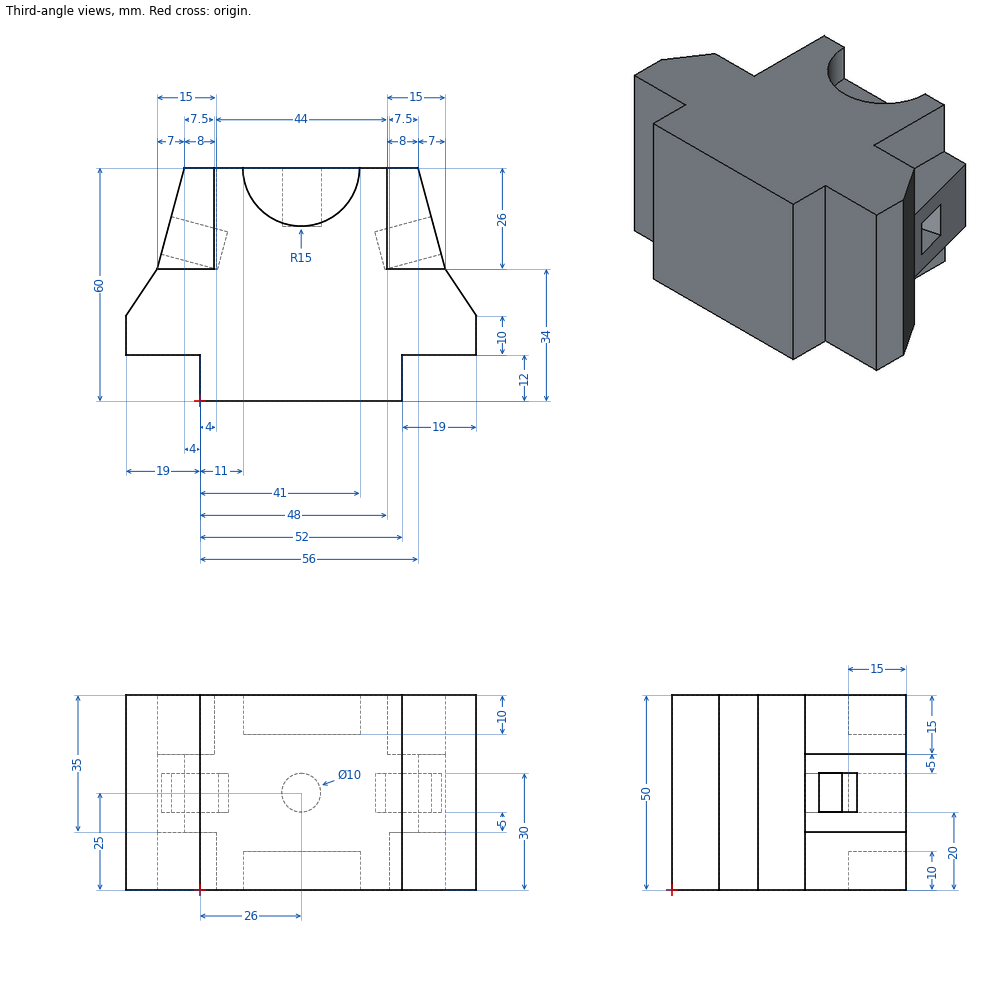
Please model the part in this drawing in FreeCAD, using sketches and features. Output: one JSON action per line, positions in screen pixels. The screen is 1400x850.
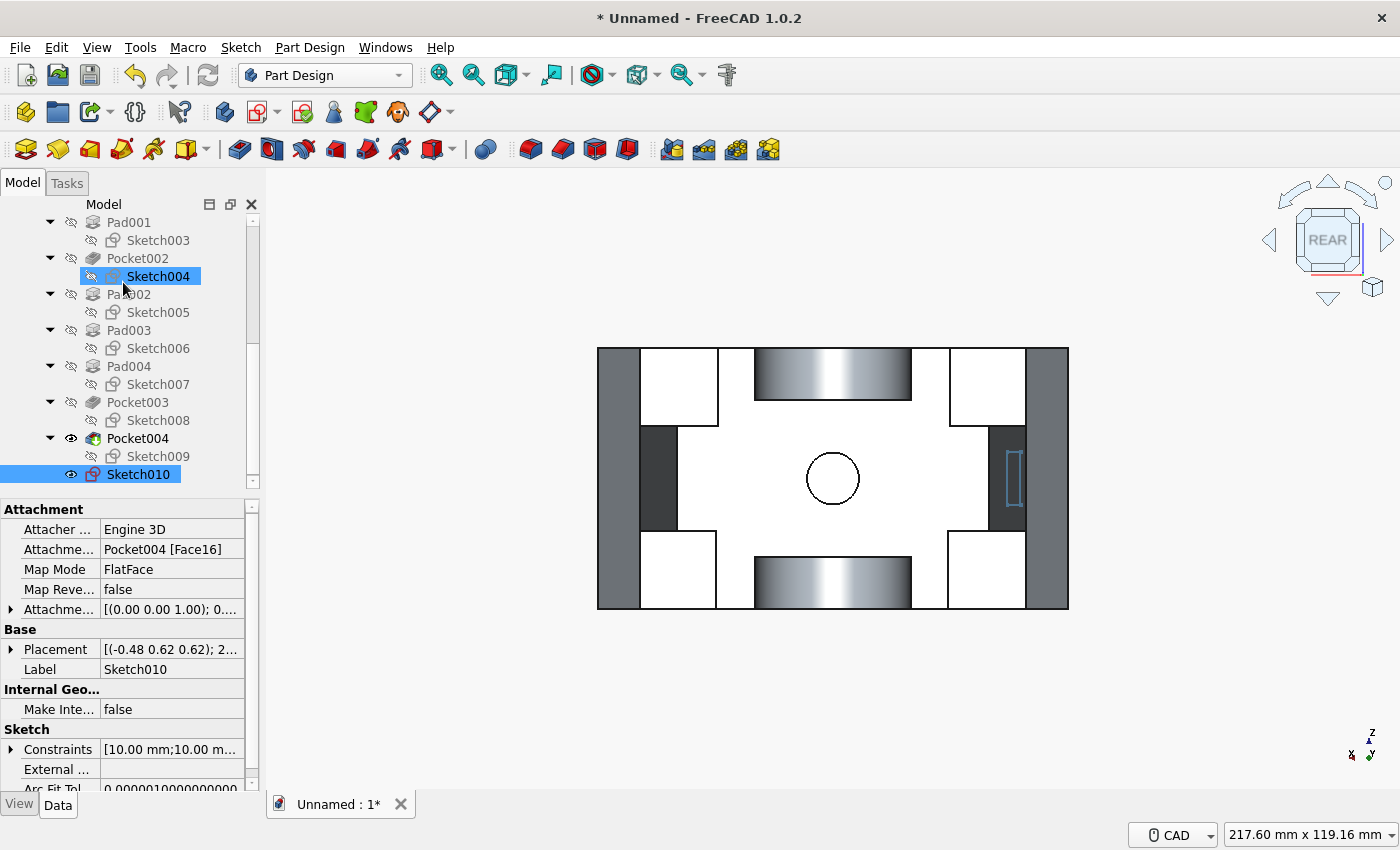
{"action": "left_click", "coordinate": [240, 150]}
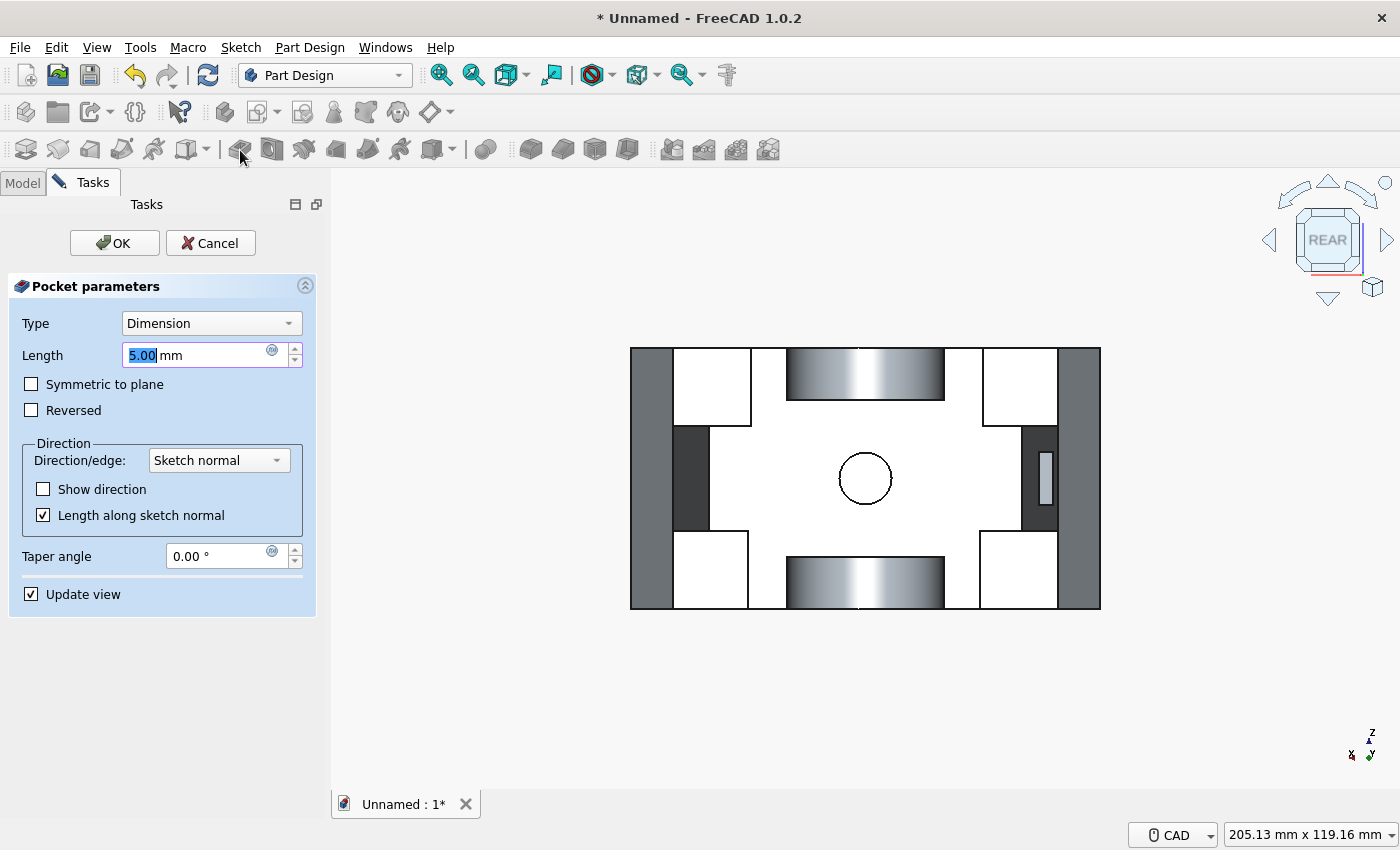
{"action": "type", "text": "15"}
{"action": "key", "text": "Tab"}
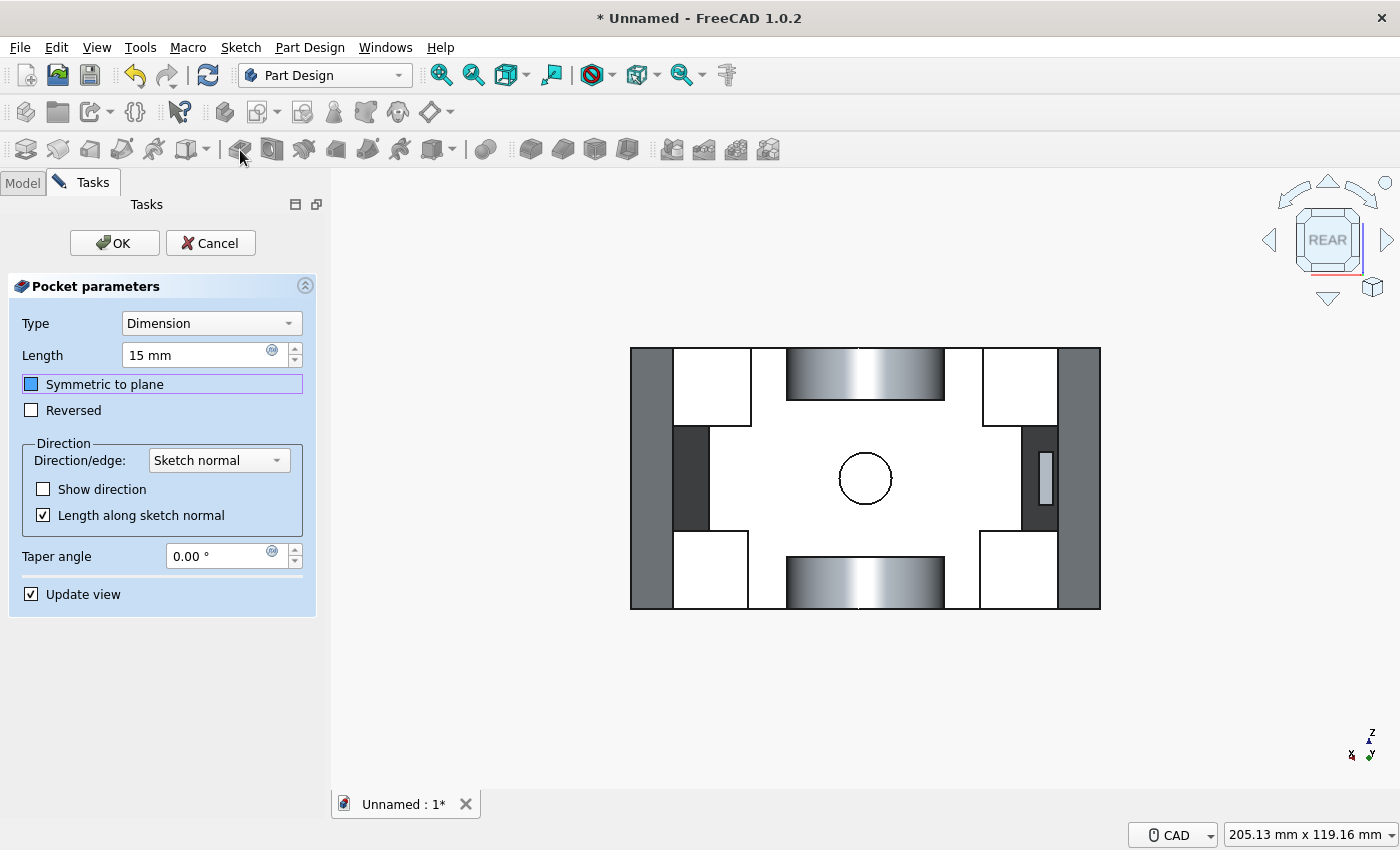
{"action": "left_click", "coordinate": [115, 243]}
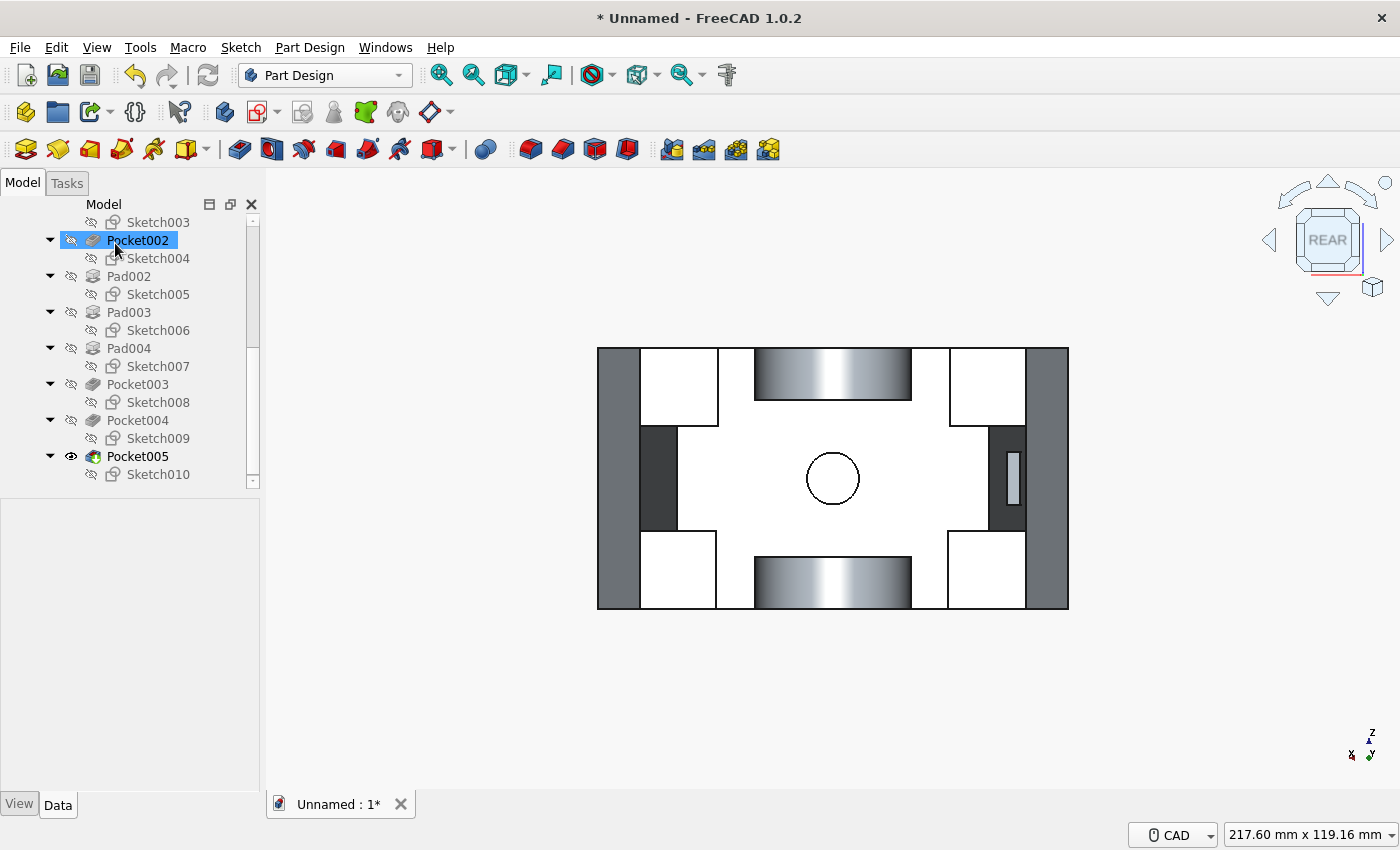
{"action": "left_click", "coordinate": [442, 76]}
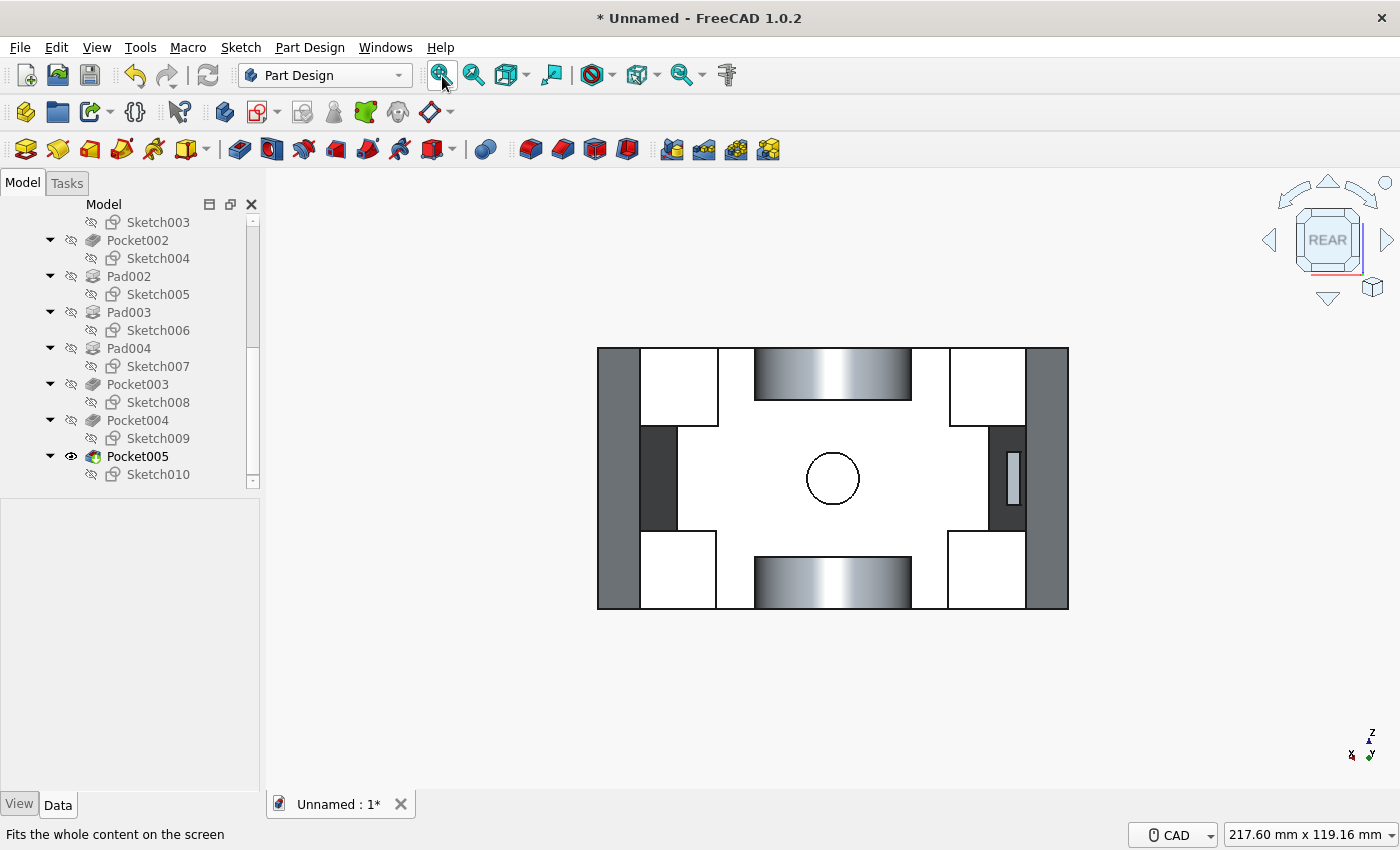
{"action": "left_click", "coordinate": [658, 477]}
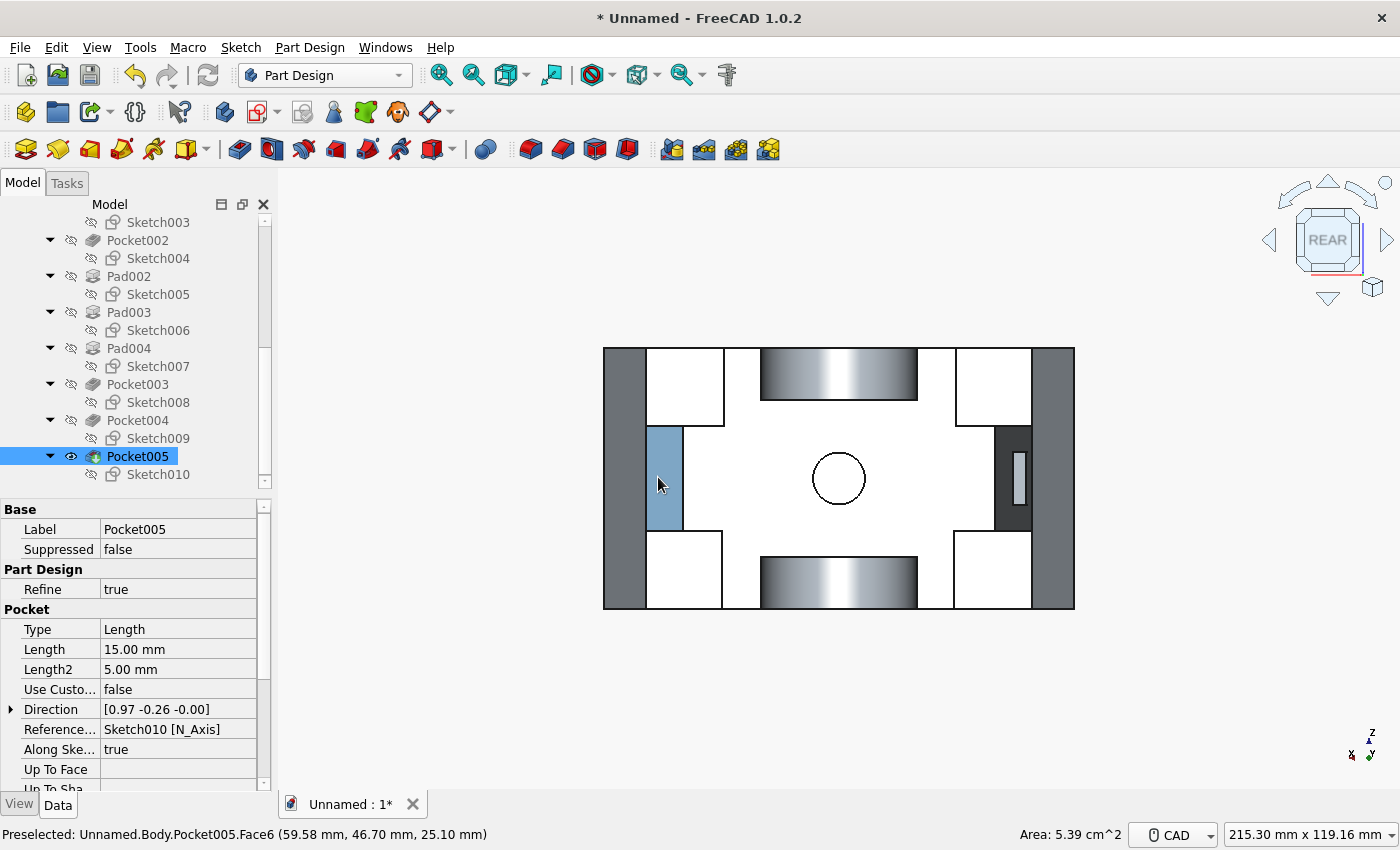
{"action": "left_click", "coordinate": [258, 112]}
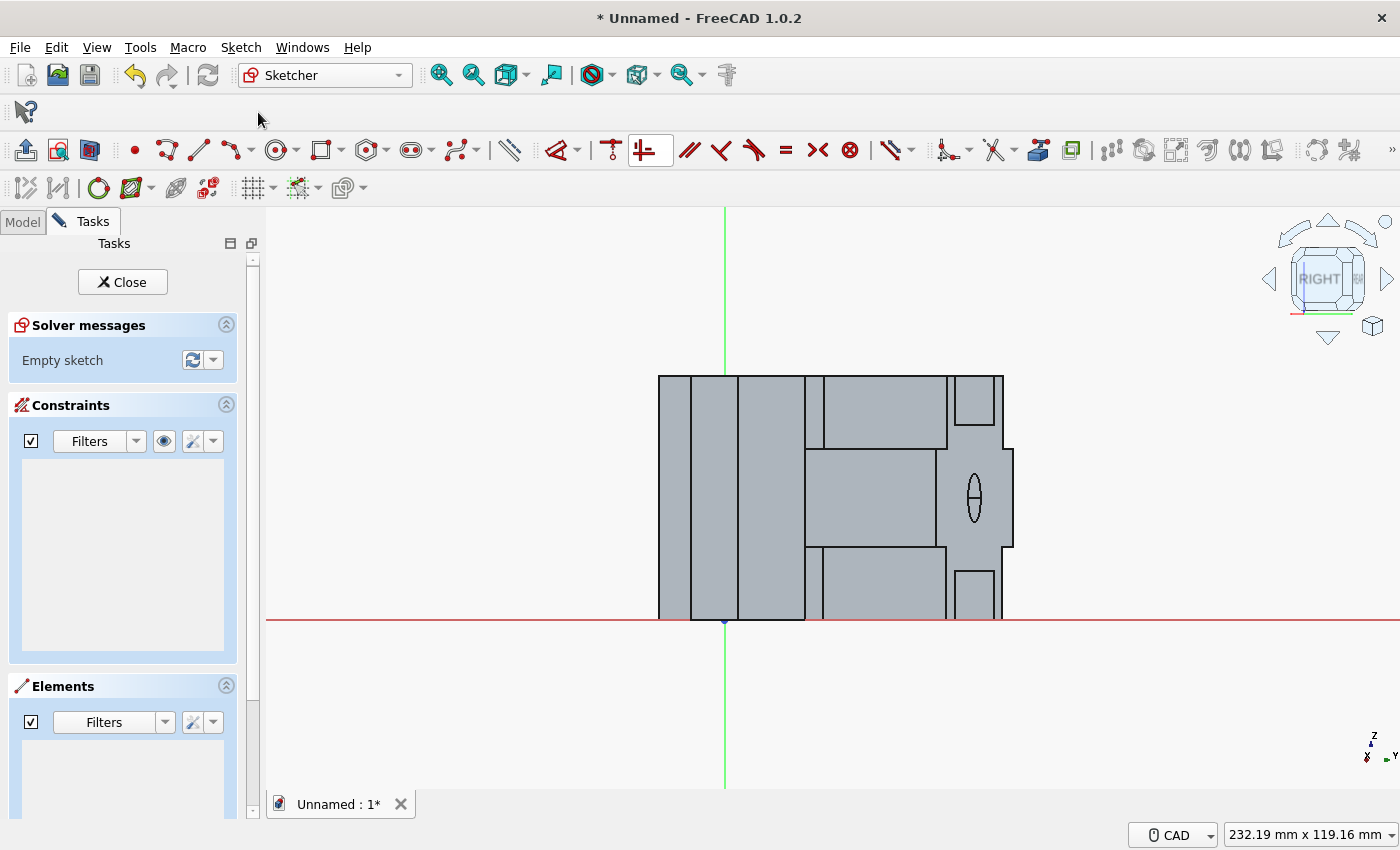
{"action": "left_click", "coordinate": [90, 150]}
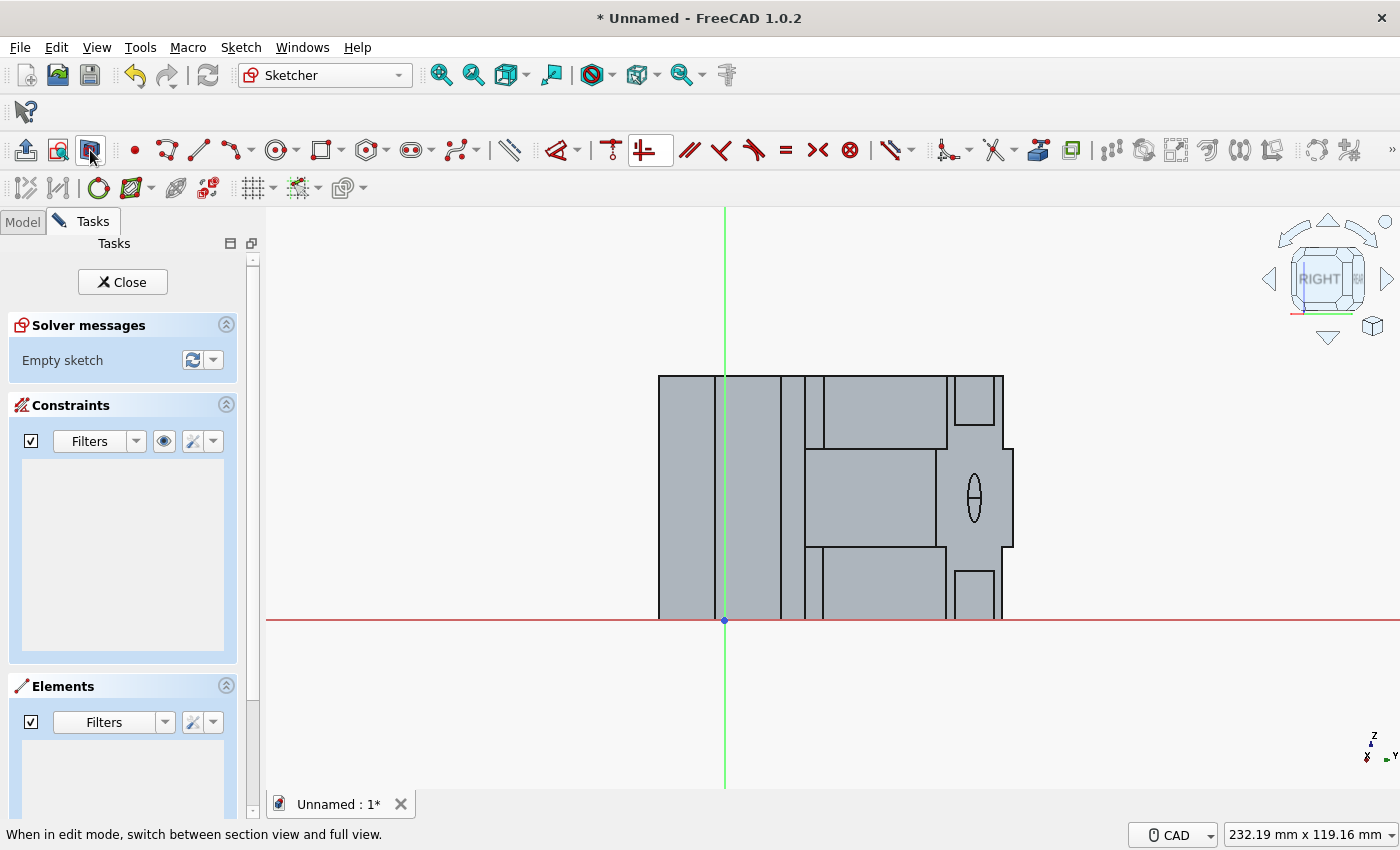
{"action": "scroll", "coordinate": [862, 498], "scroll_direction": "up", "scroll_amount": 10}